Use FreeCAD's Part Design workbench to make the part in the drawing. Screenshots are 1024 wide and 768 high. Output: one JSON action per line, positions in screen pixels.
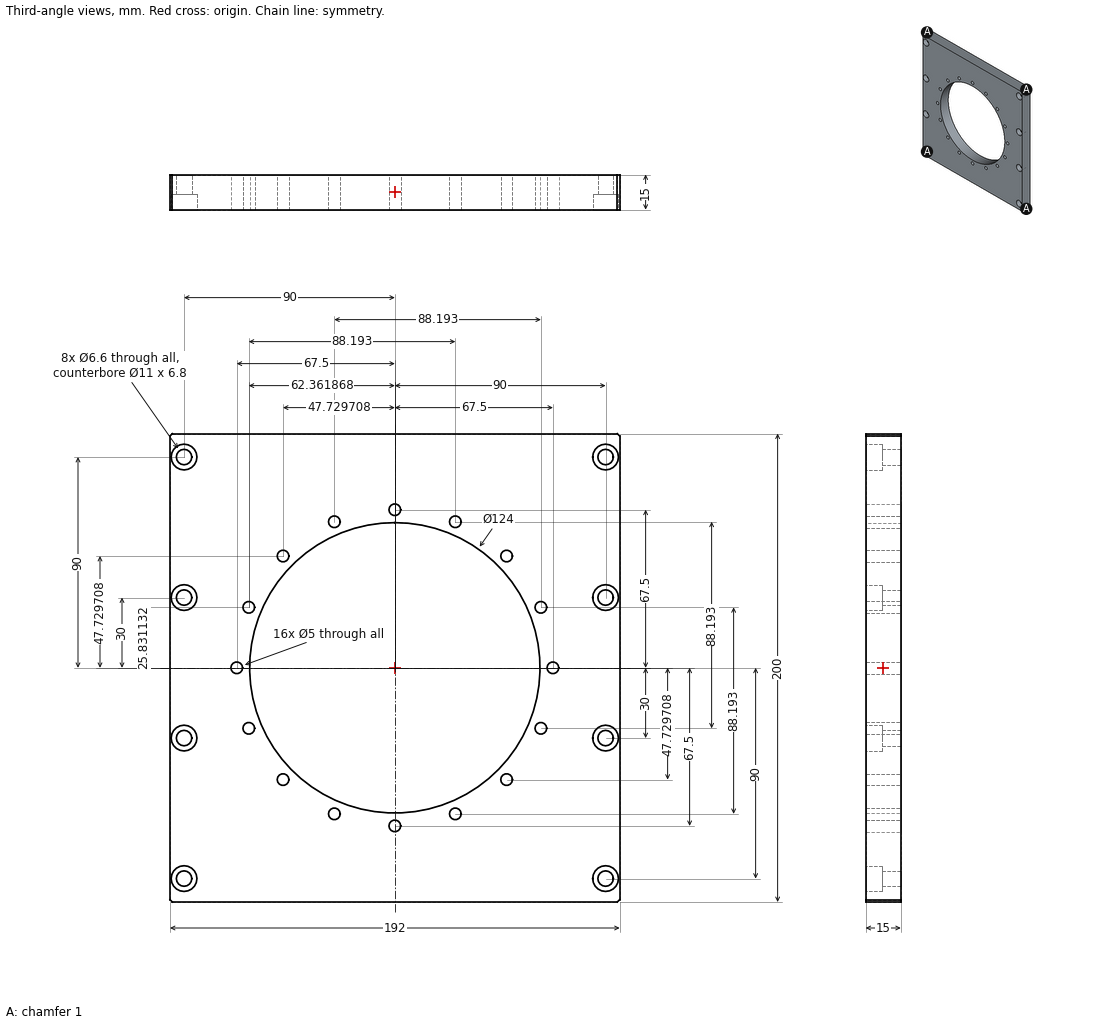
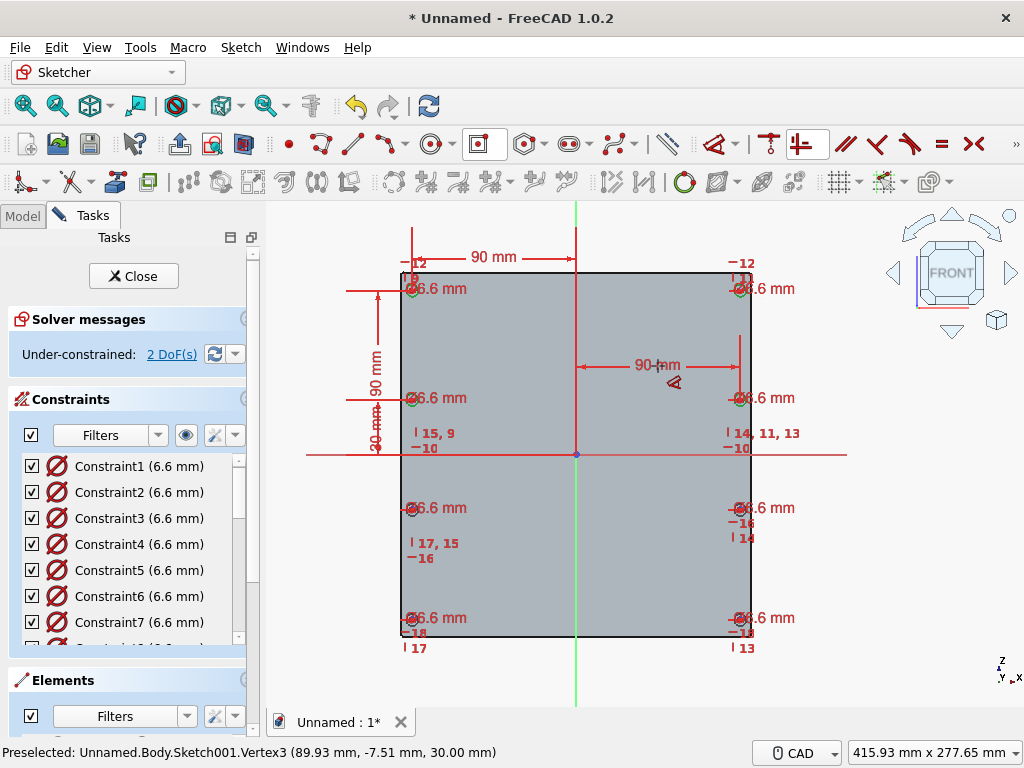
{"action": "left_click", "coordinate": [740, 620]}
{"action": "left_click", "coordinate": [774, 537]}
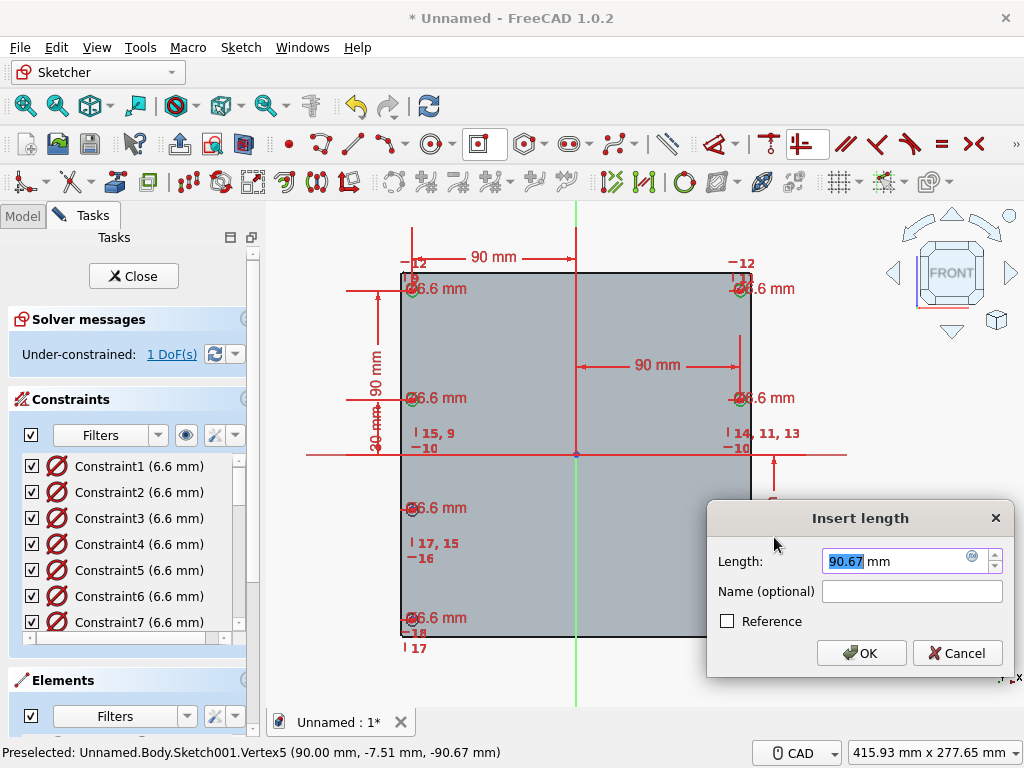
{"action": "type", "text": "90"}
{"action": "key", "text": "Return"}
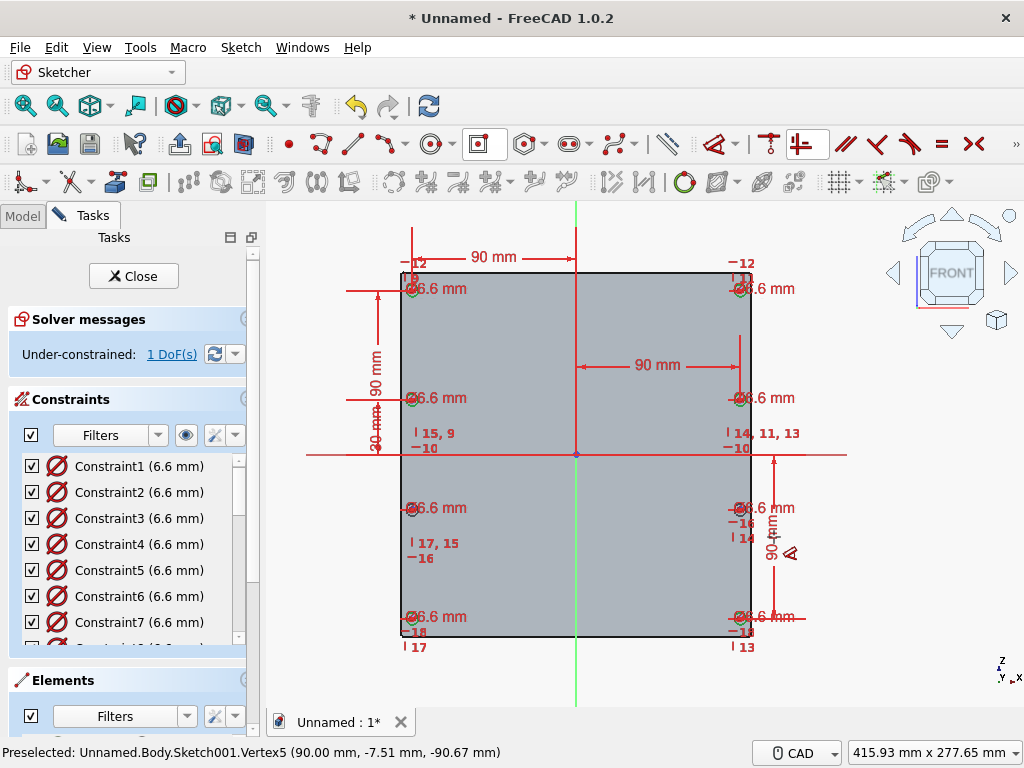
{"action": "left_click", "coordinate": [740, 510]}
{"action": "left_click", "coordinate": [774, 482]}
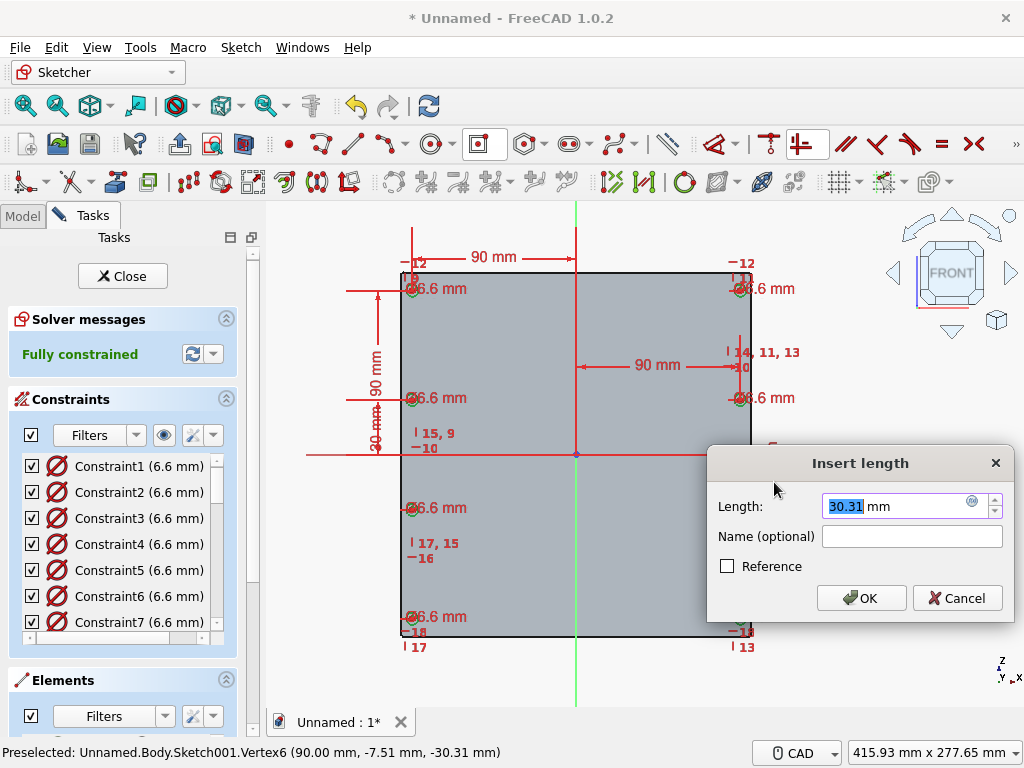
{"action": "type", "text": "30"}
{"action": "key", "text": "Return"}
{"action": "key", "text": "Escape"}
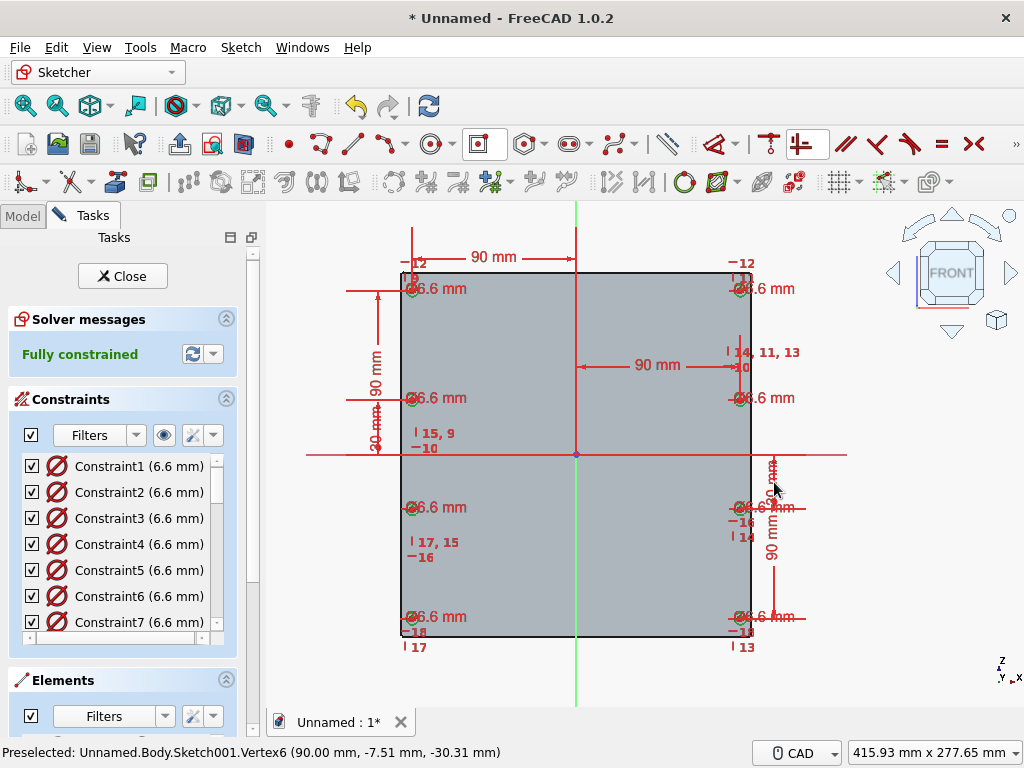
{"action": "left_click", "coordinate": [123, 276]}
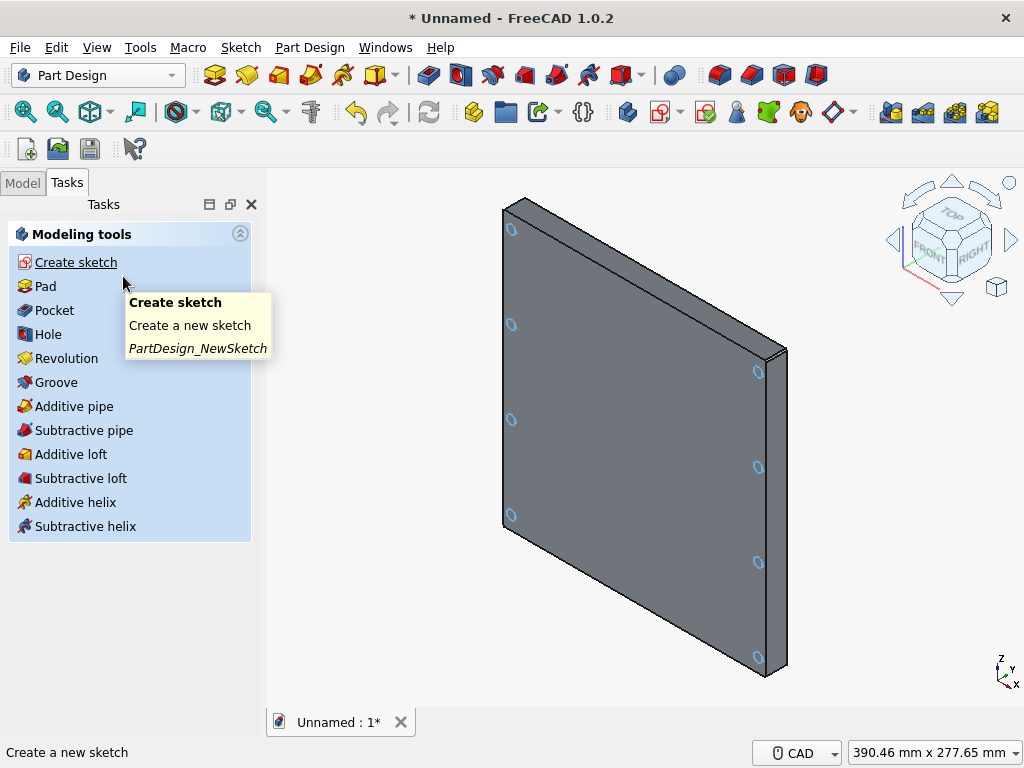
{"action": "left_click", "coordinate": [462, 76]}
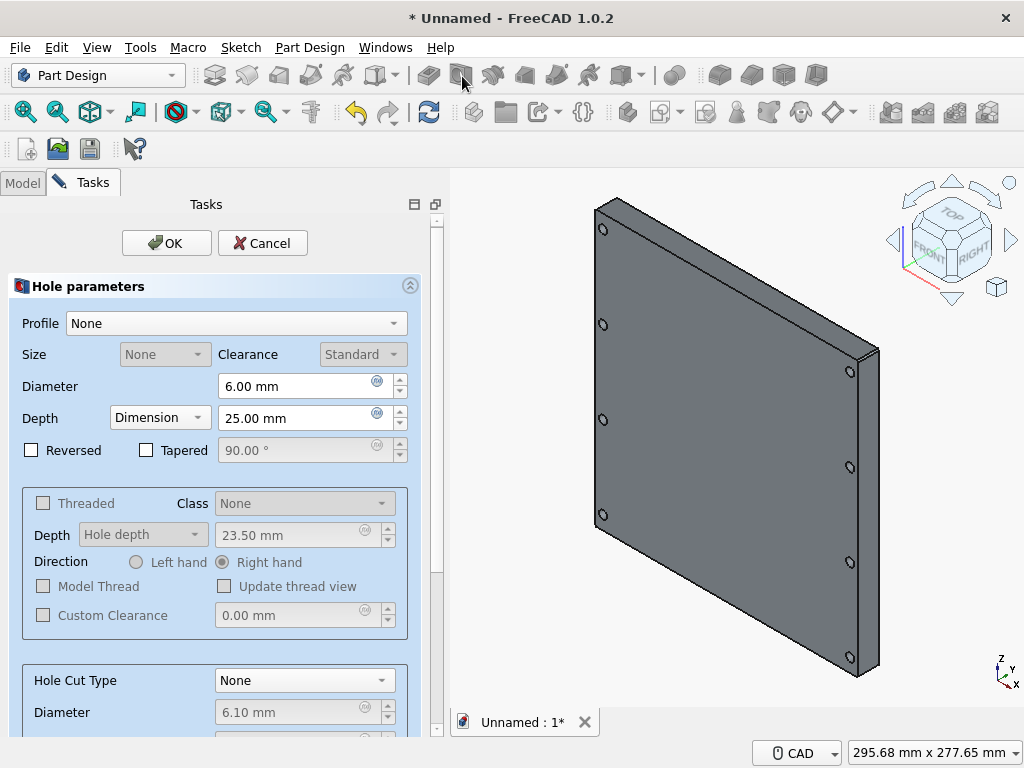
{"action": "triple_click", "coordinate": [305, 386]}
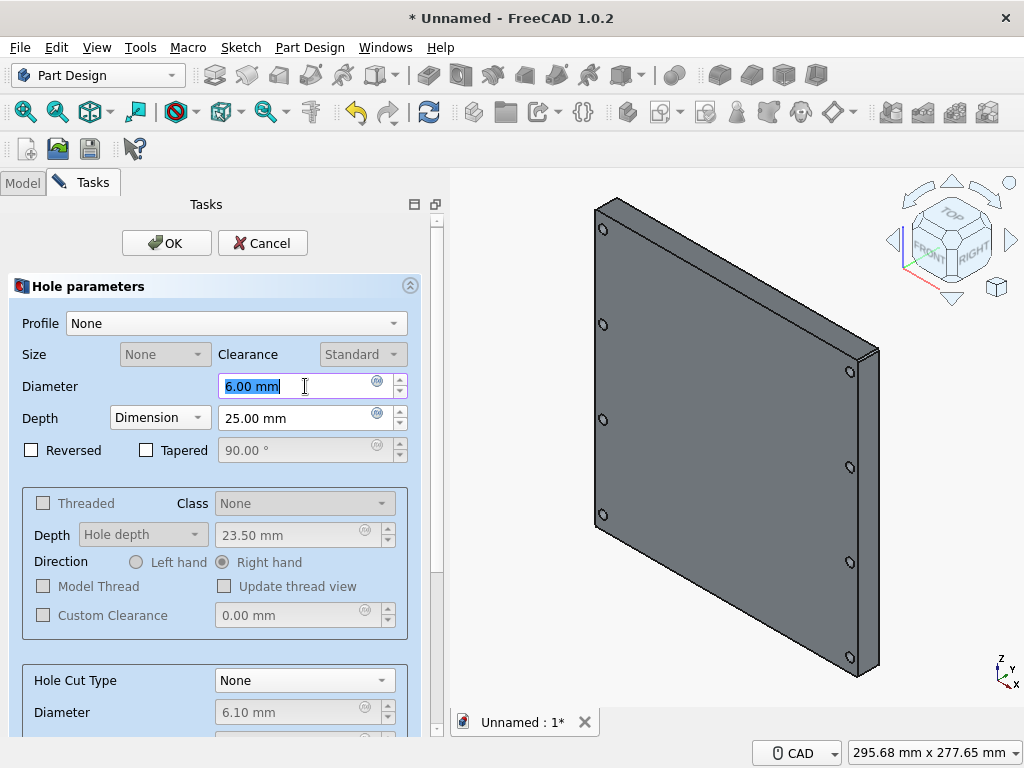
{"action": "type", "text": "6.6"}
{"action": "key", "text": "Tab"}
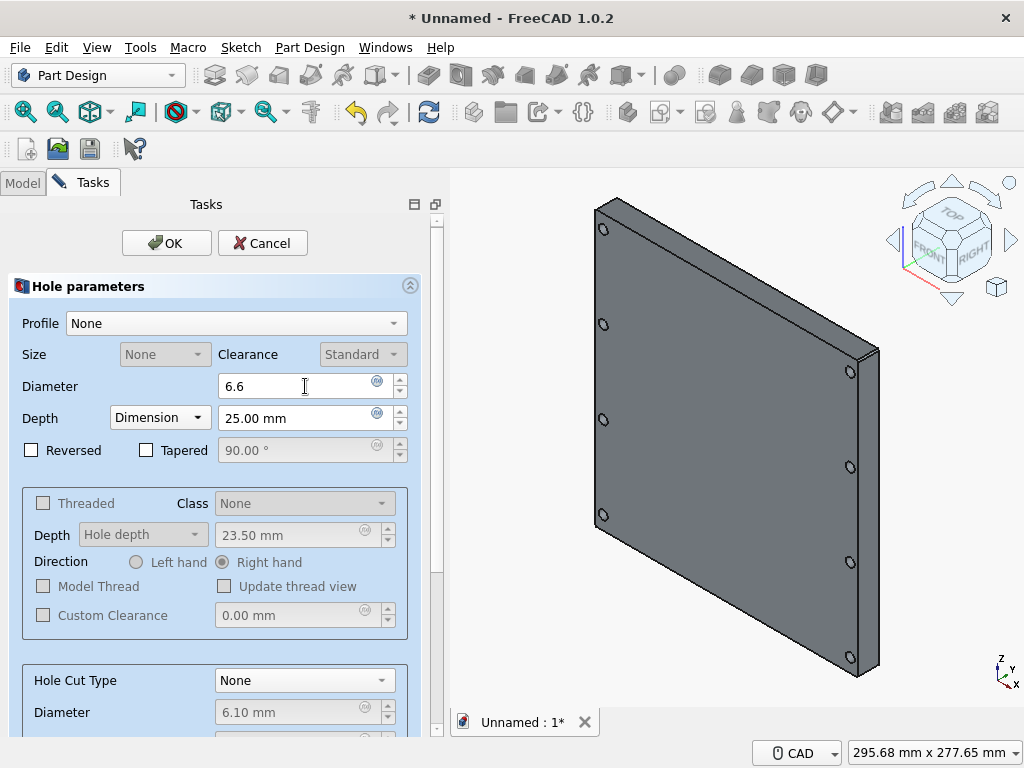
{"action": "left_click", "coordinate": [161, 418]}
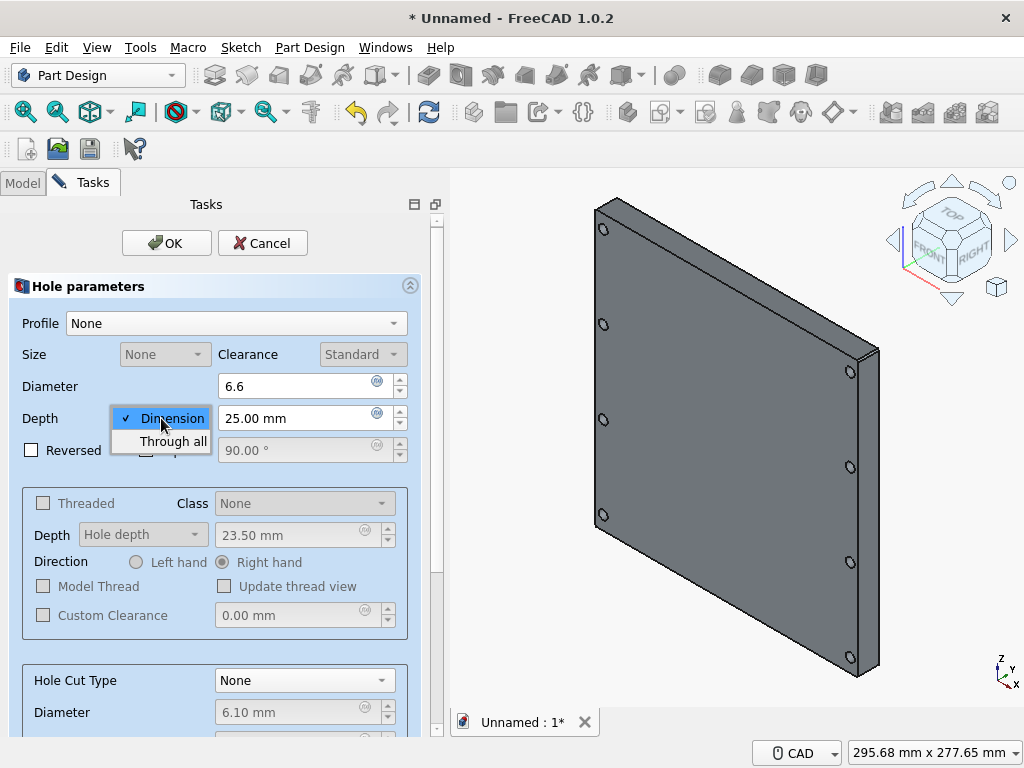
{"action": "left_click", "coordinate": [160, 442]}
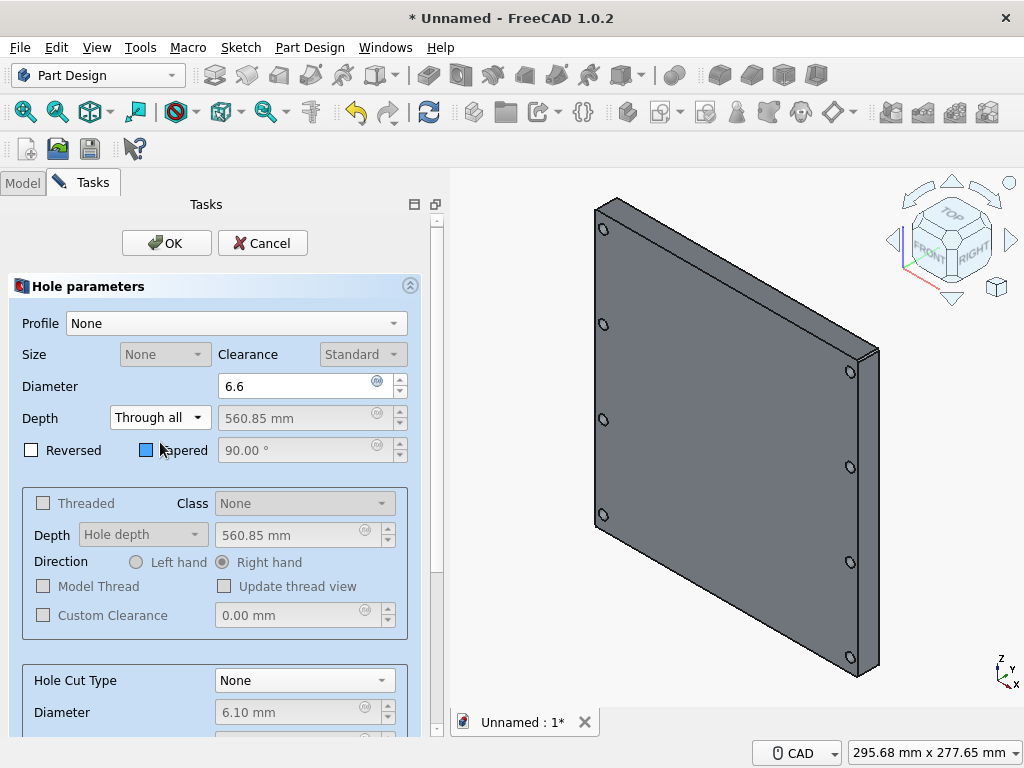
{"action": "left_click", "coordinate": [306, 680]}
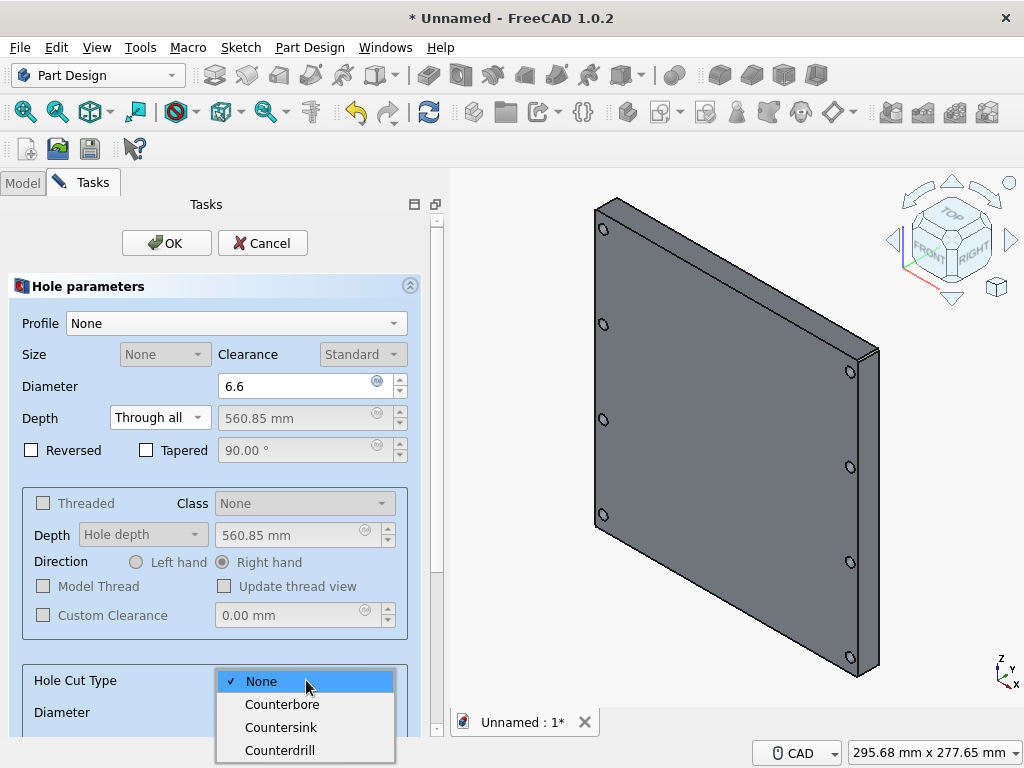
{"action": "left_click", "coordinate": [304, 704]}